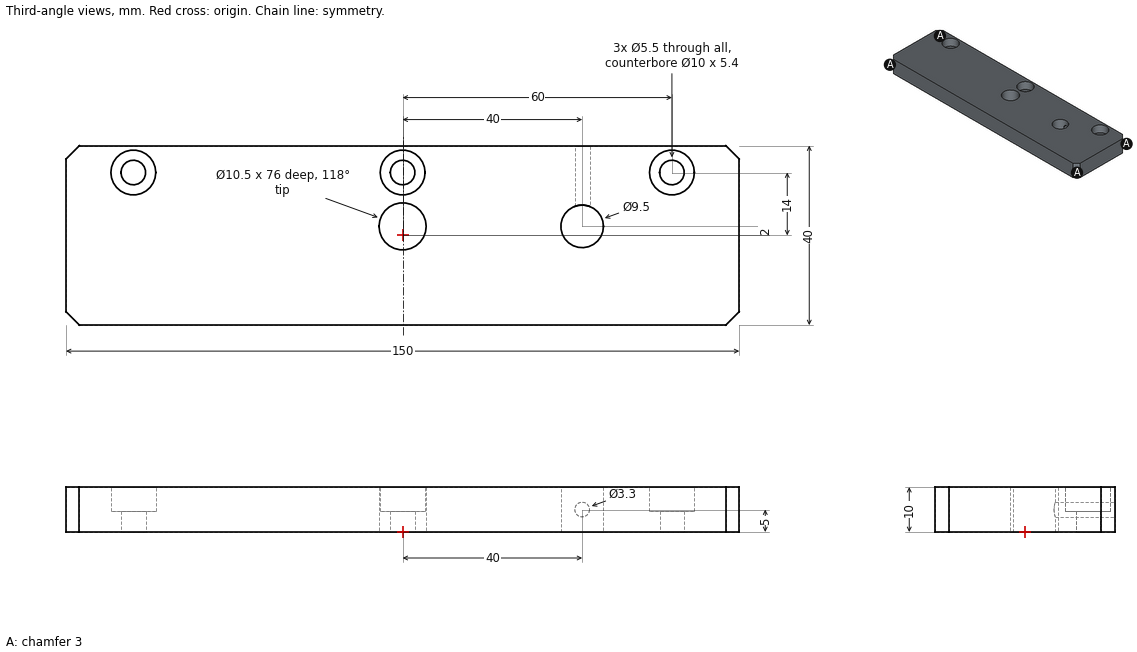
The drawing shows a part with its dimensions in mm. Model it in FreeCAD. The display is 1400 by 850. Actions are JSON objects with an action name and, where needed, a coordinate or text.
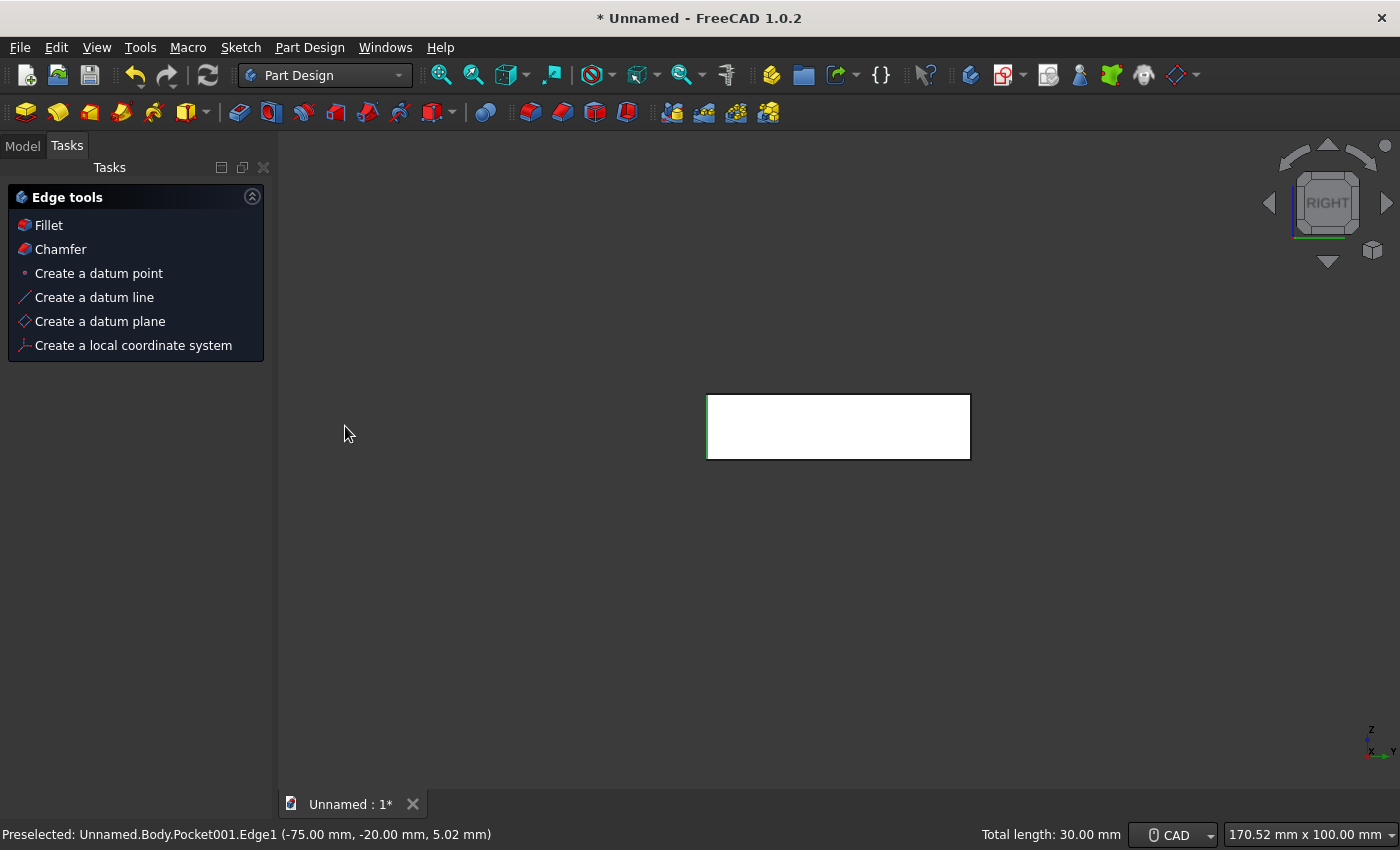
{"action": "left_click", "coordinate": [442, 76]}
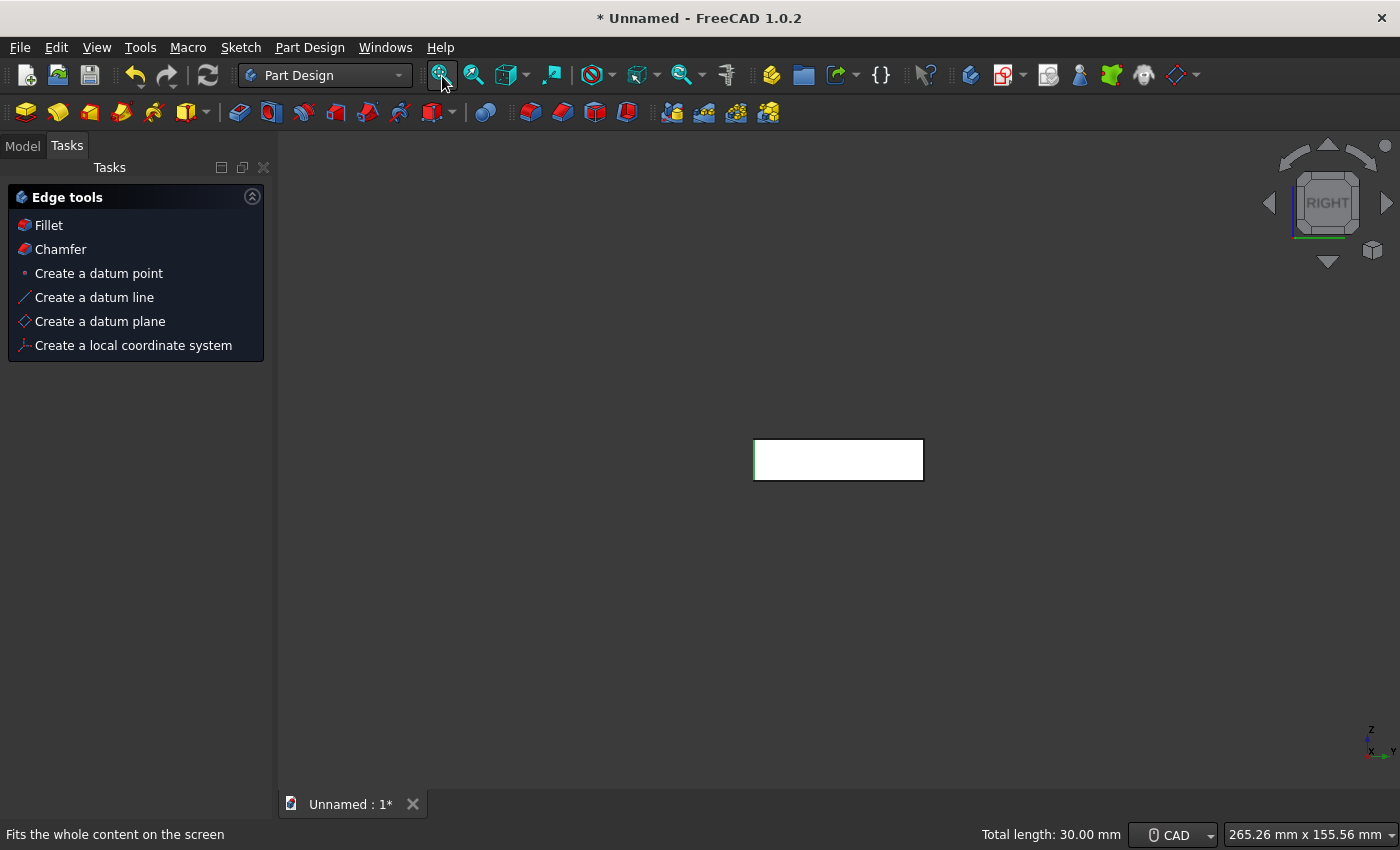
{"action": "left_click", "coordinate": [924, 459], "text": "ctrl"}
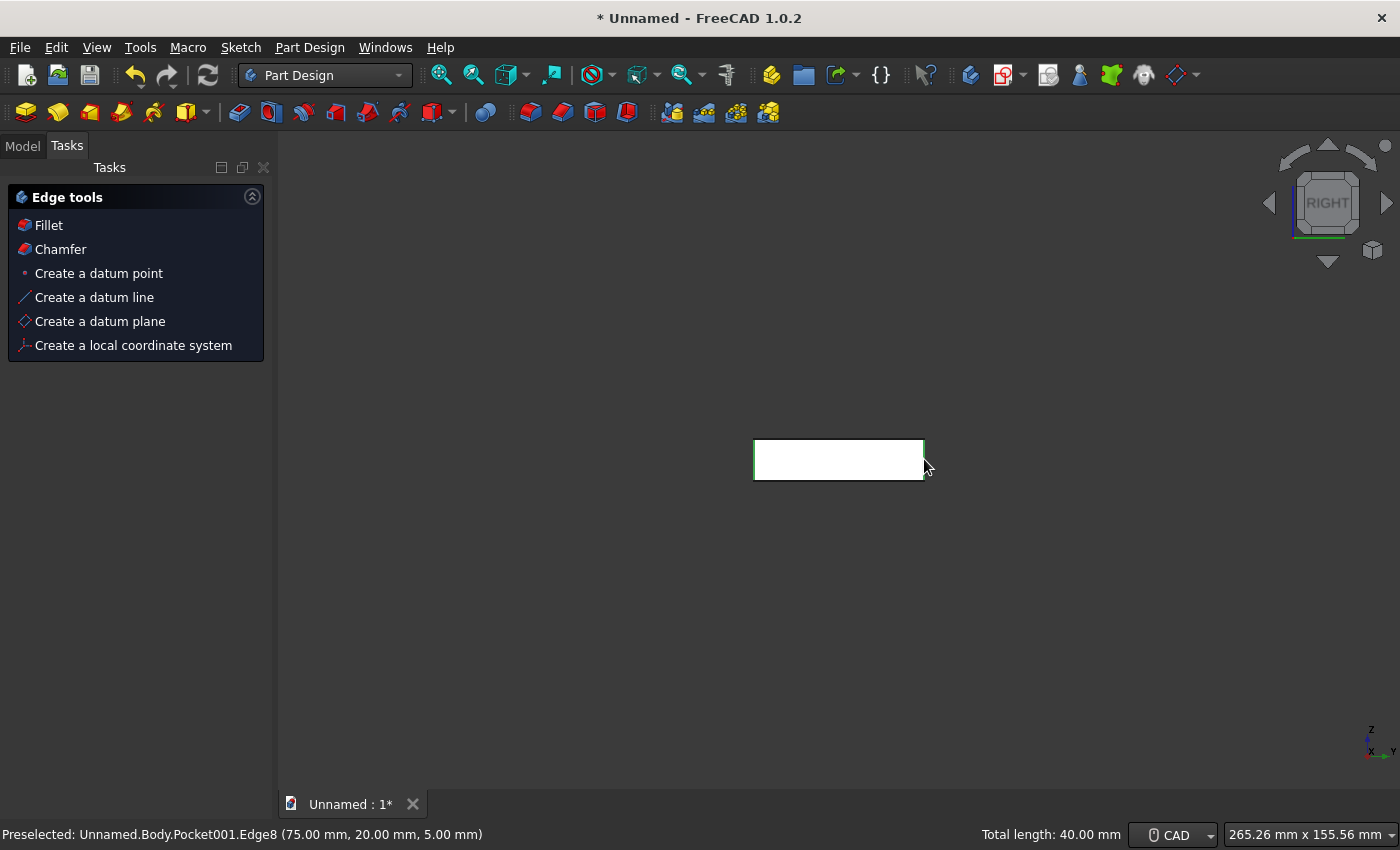
{"action": "left_click", "coordinate": [564, 112]}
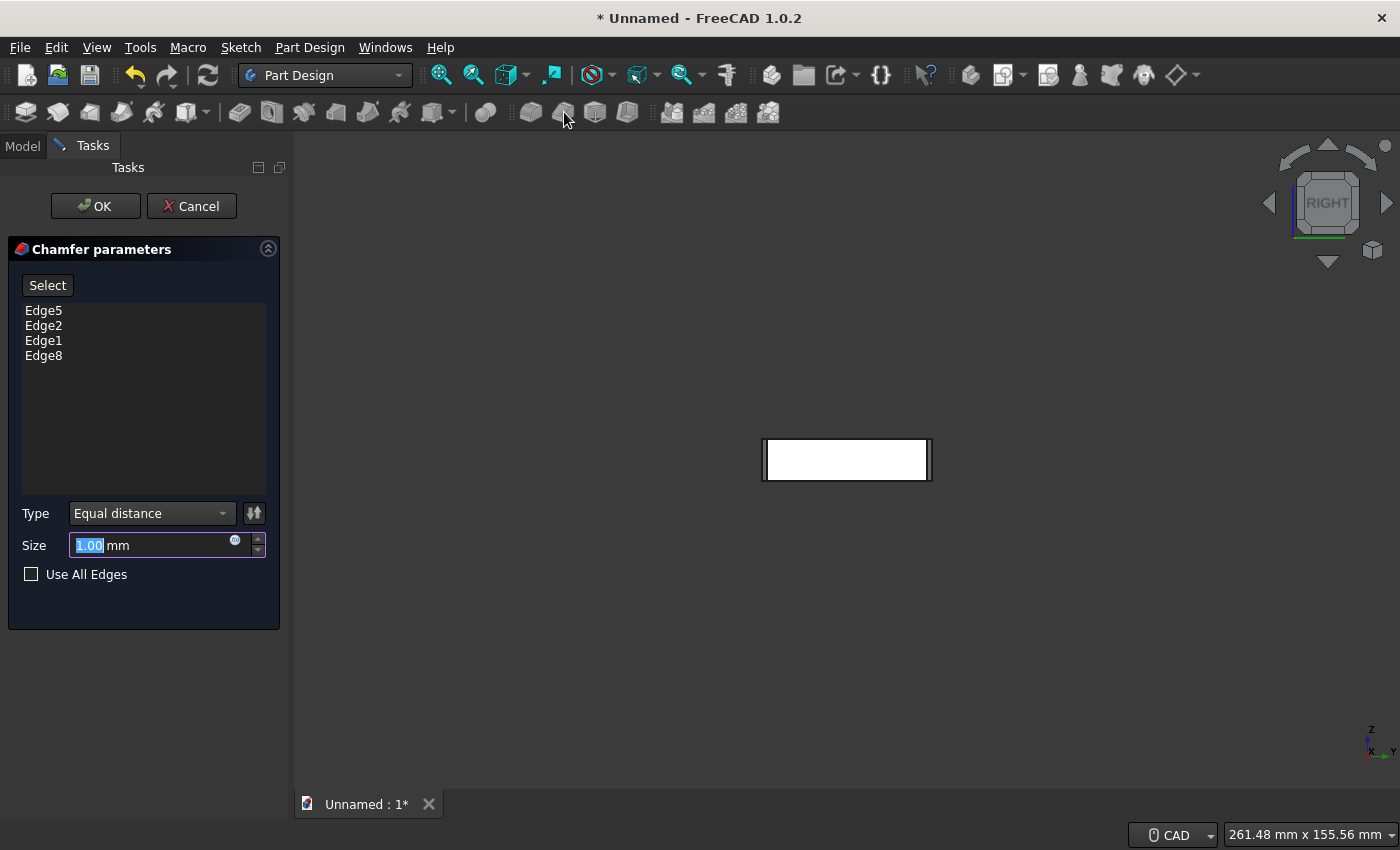
{"action": "type", "text": "3"}
{"action": "key", "text": "Tab"}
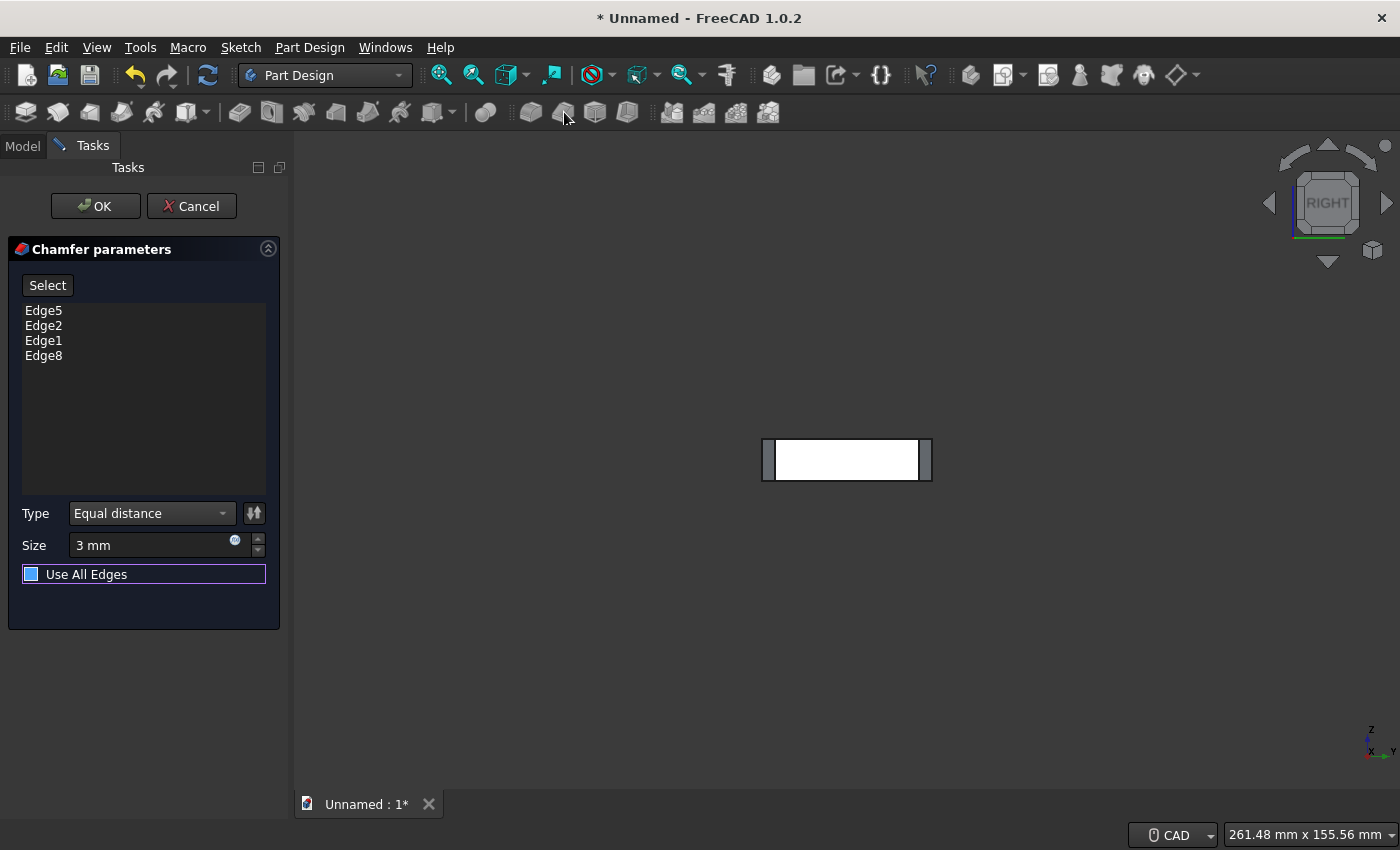
{"action": "left_click", "coordinate": [96, 206]}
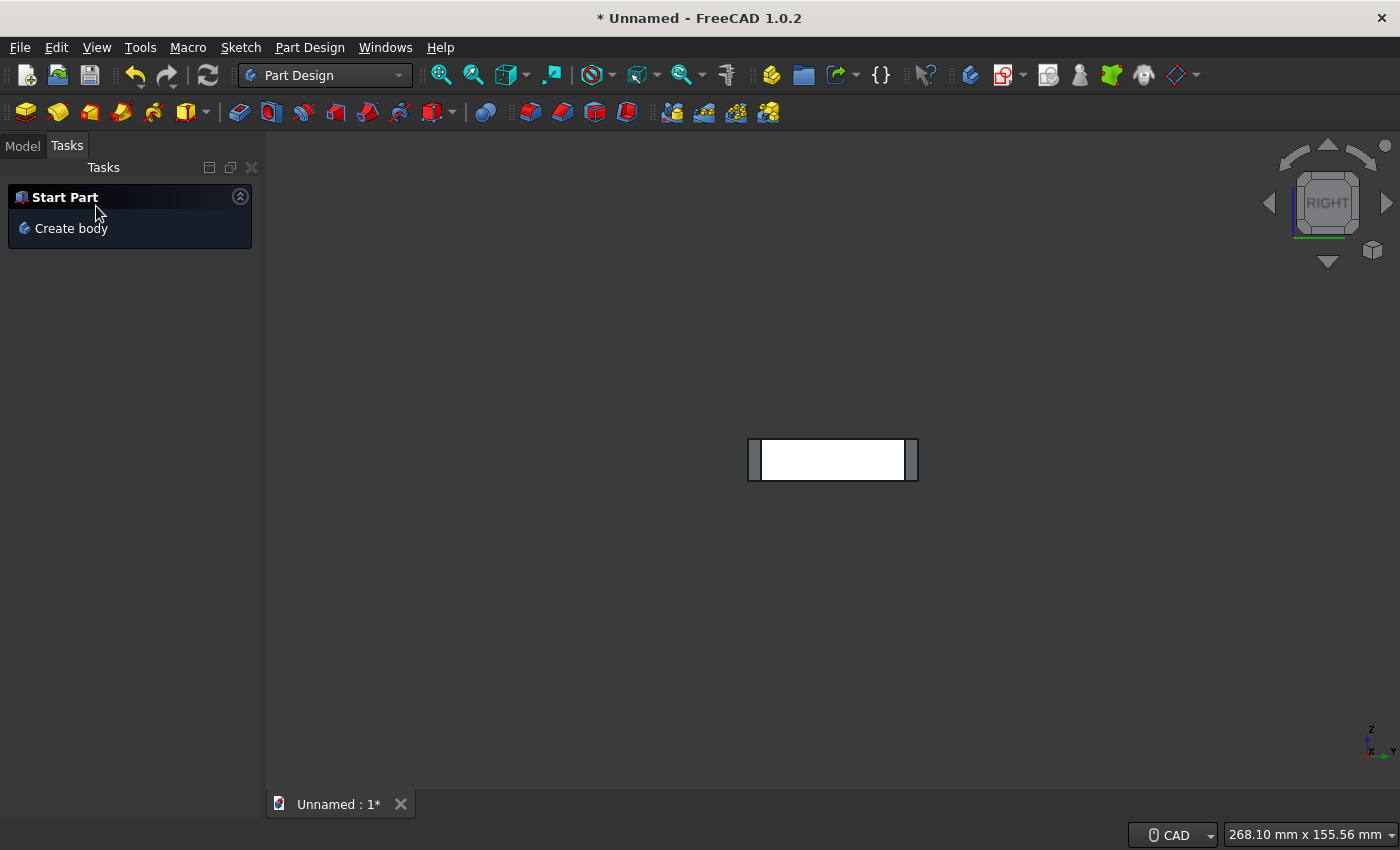
{"action": "key", "text": "0"}